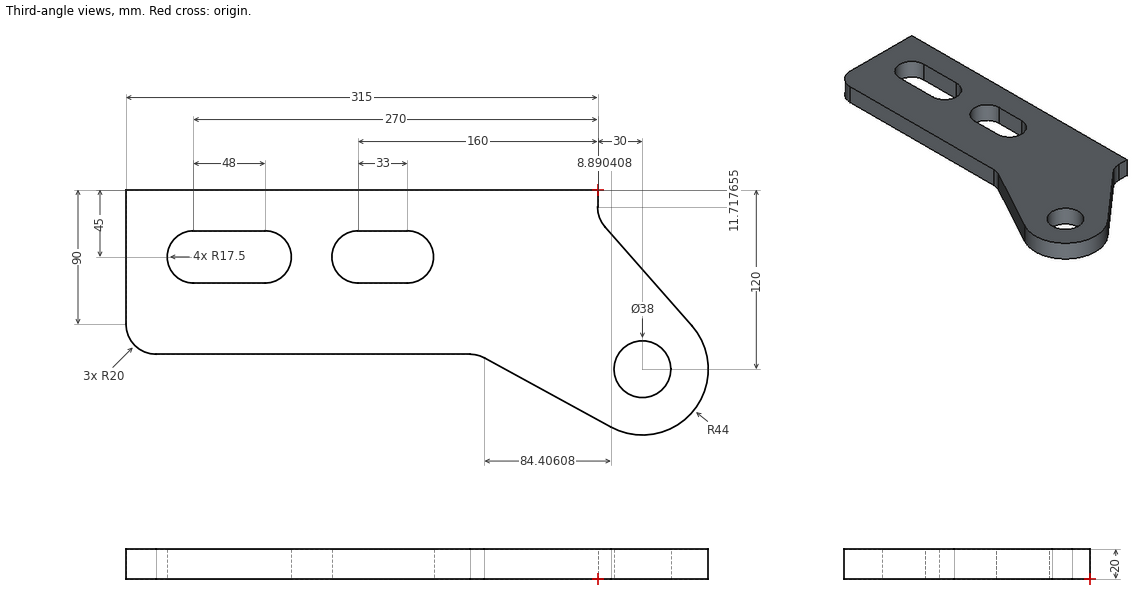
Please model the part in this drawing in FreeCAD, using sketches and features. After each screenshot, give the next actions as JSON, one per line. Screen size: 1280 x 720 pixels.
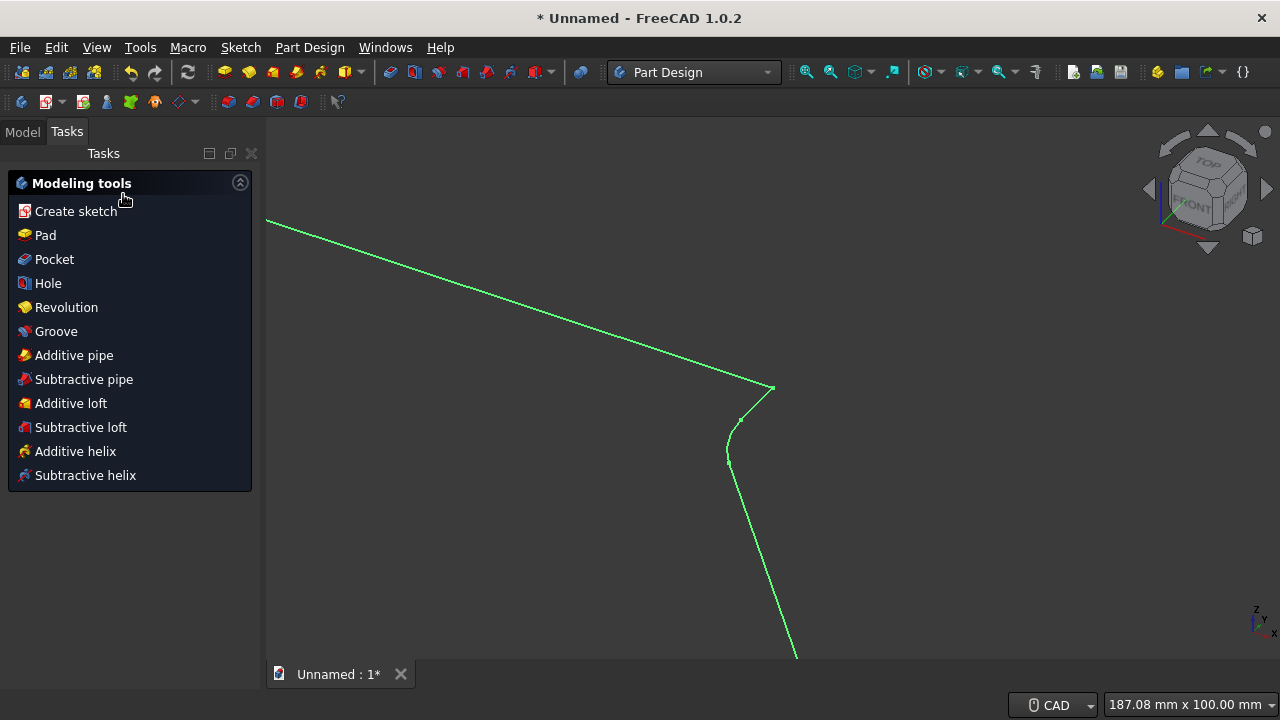
{"action": "left_click", "coordinate": [226, 72]}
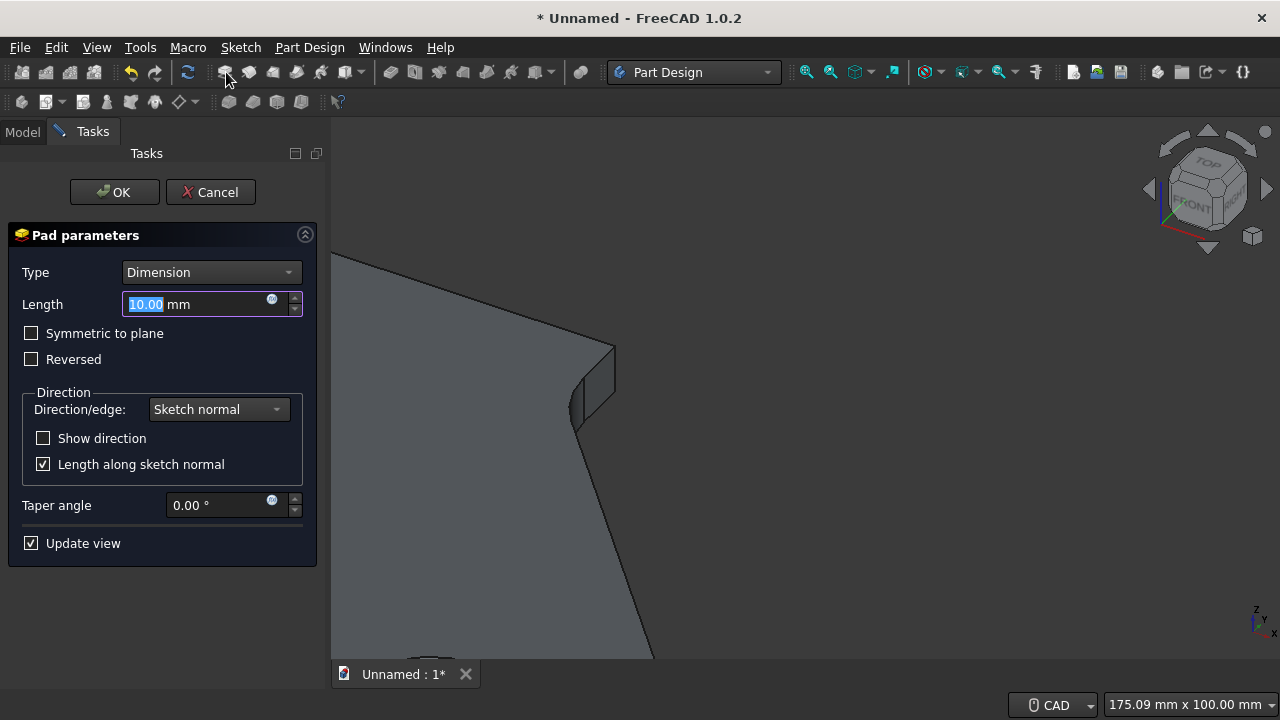
{"action": "type", "text": "20"}
{"action": "key", "text": "Tab"}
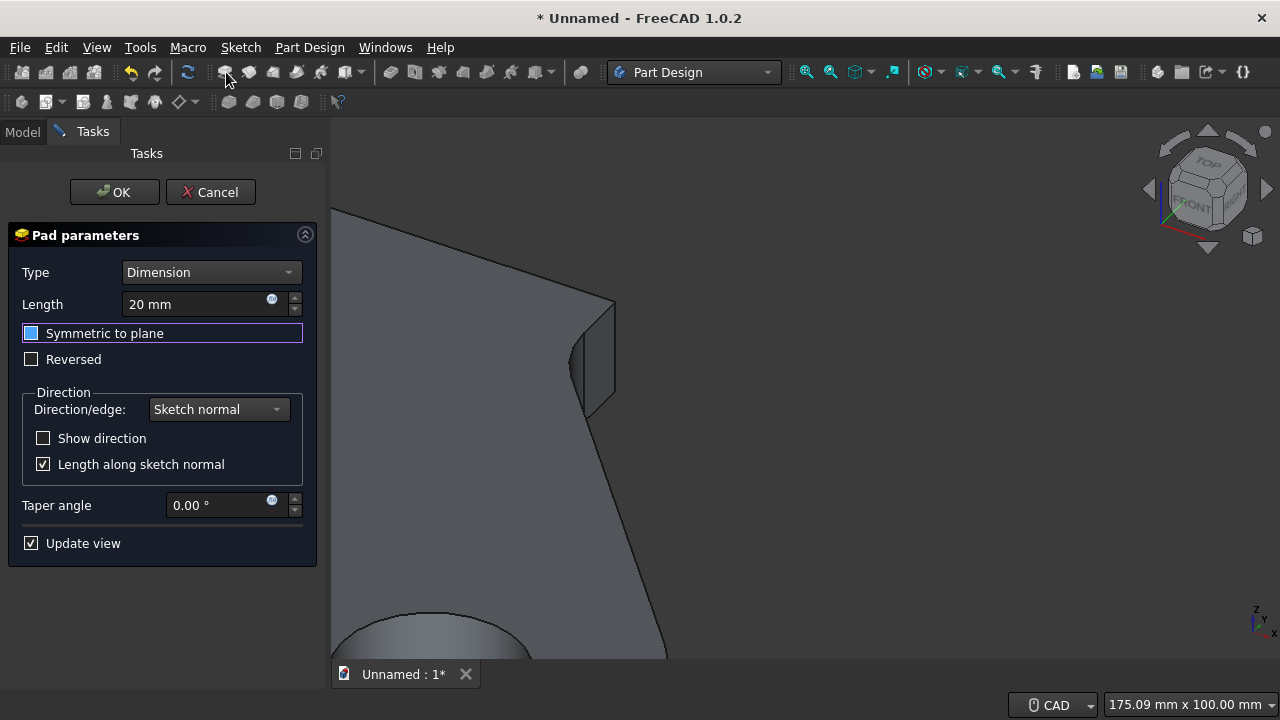
{"action": "left_click", "coordinate": [115, 192]}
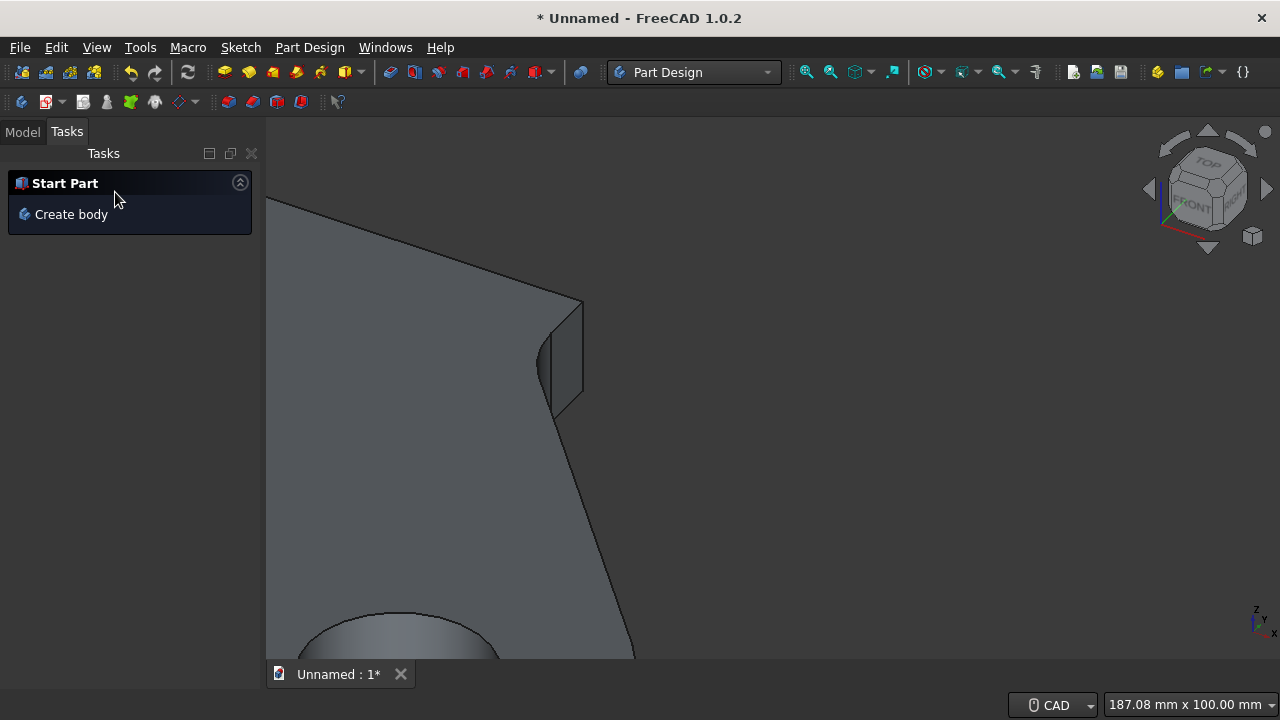
{"action": "key", "text": "0"}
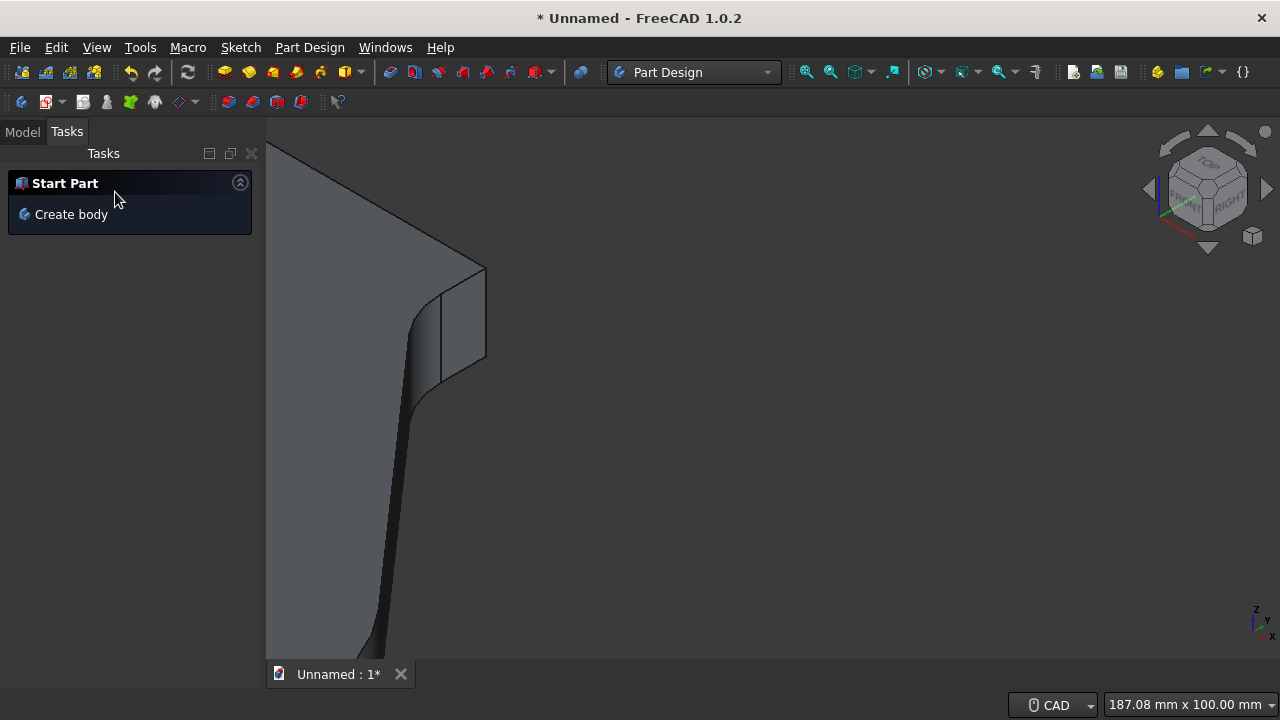
{"action": "left_click", "coordinate": [808, 72]}